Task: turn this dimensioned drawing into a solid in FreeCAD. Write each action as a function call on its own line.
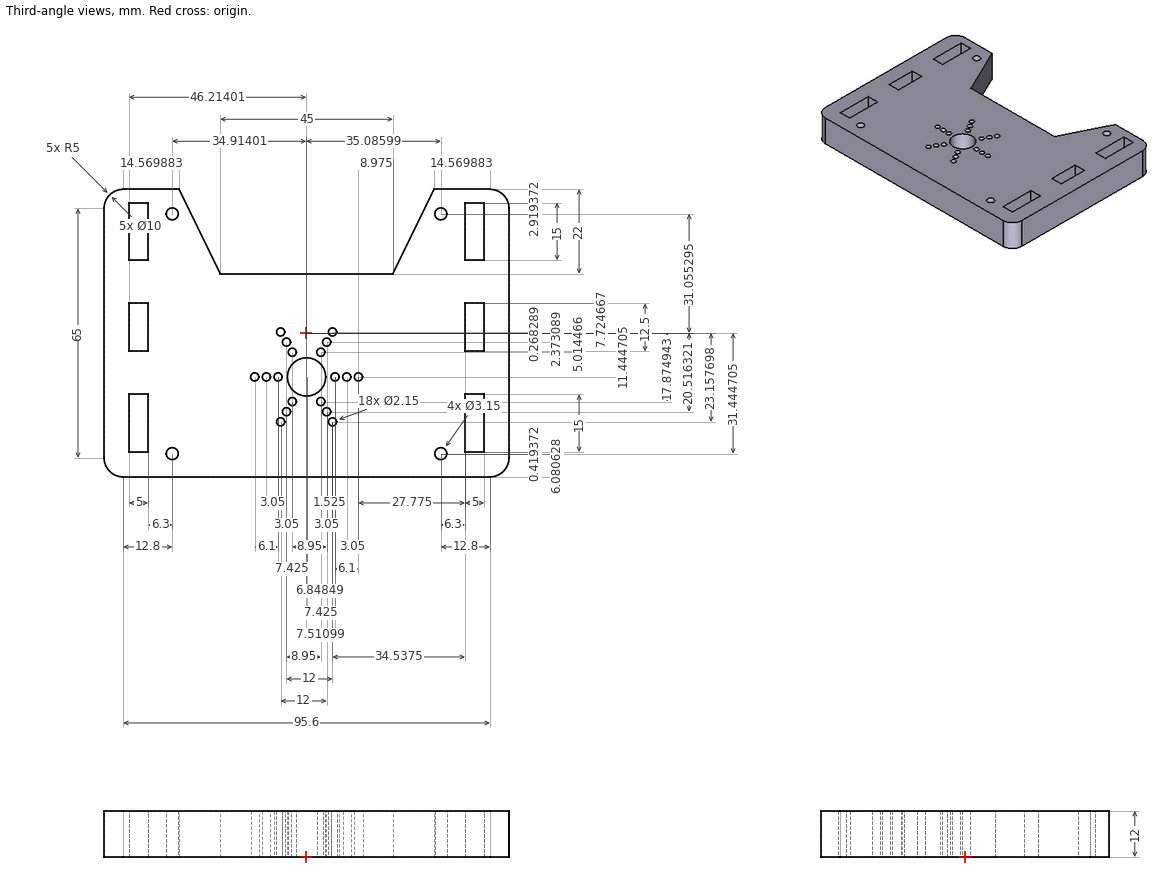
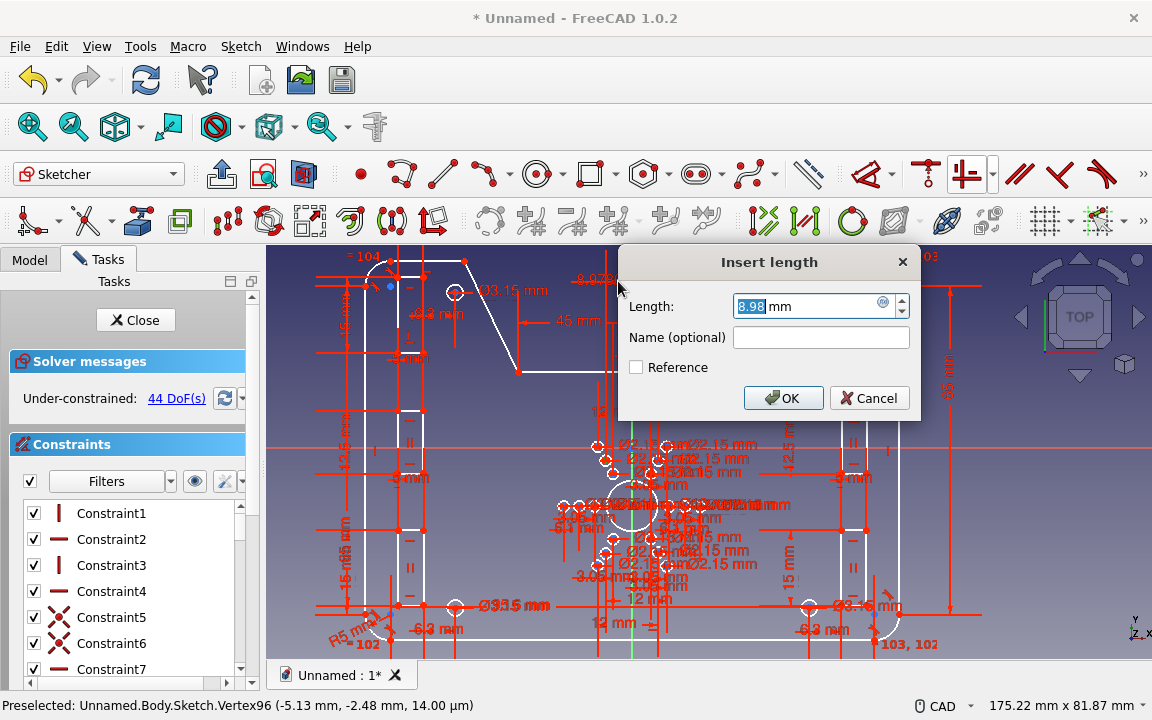
text(8.95)
key(Return)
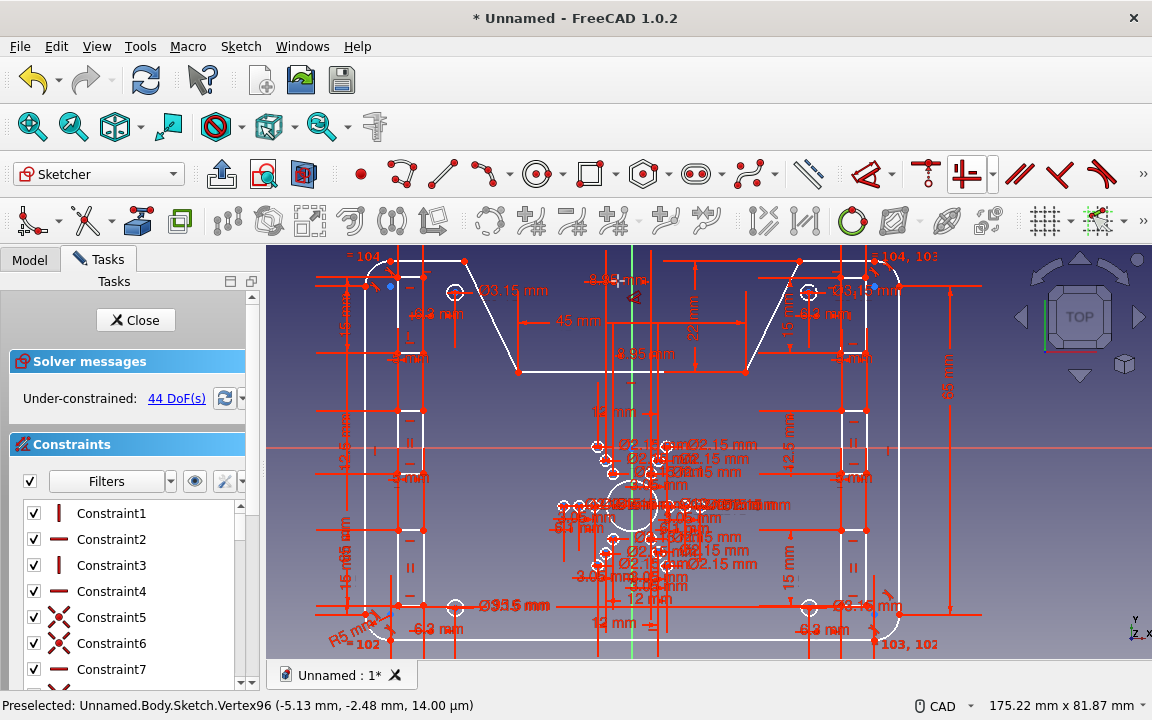
scroll(667, 566, up, 9)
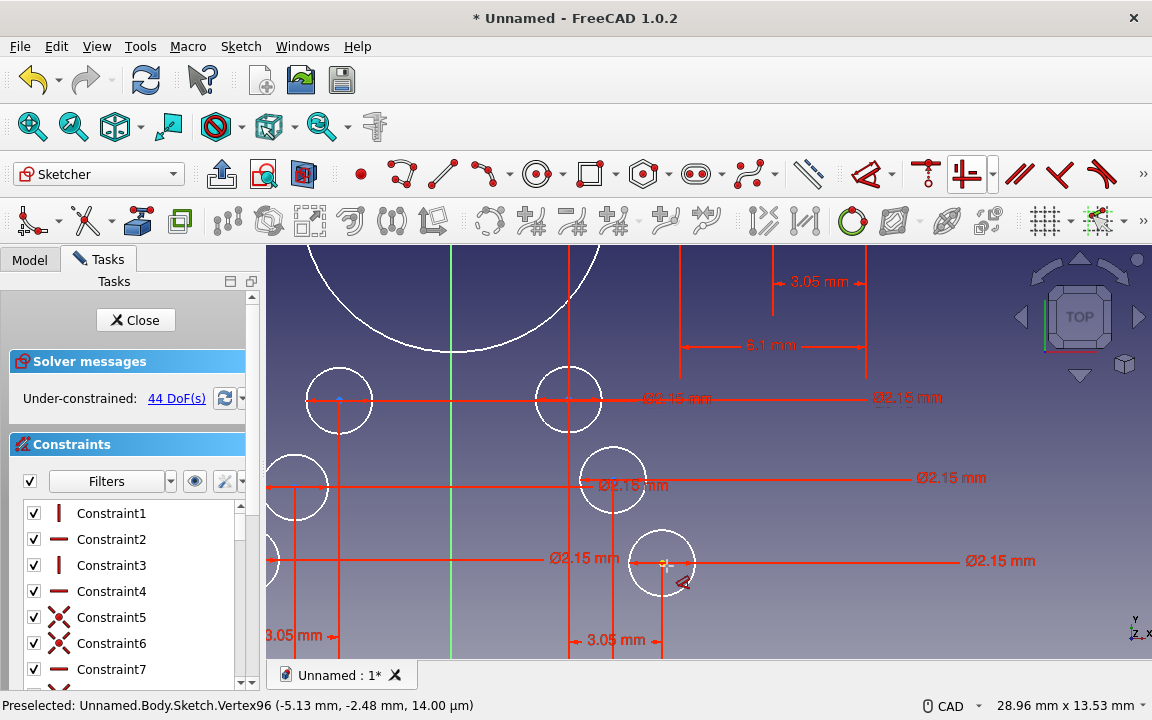
click(662, 563)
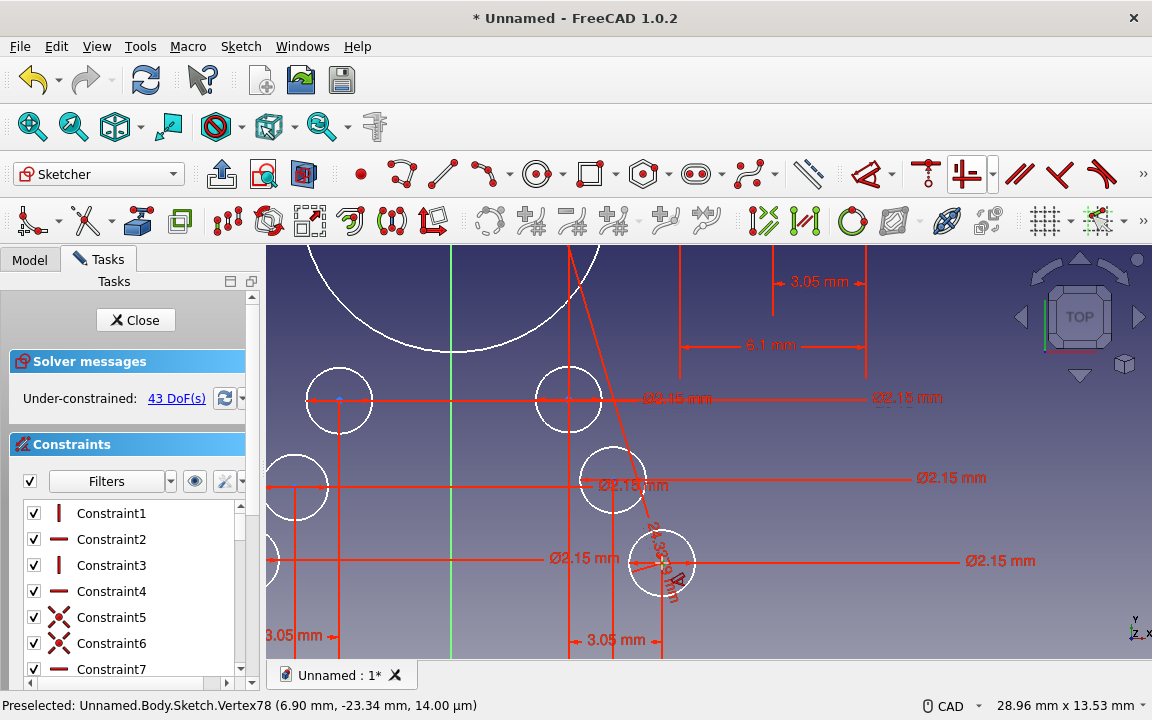
click(613, 480)
click(626, 597)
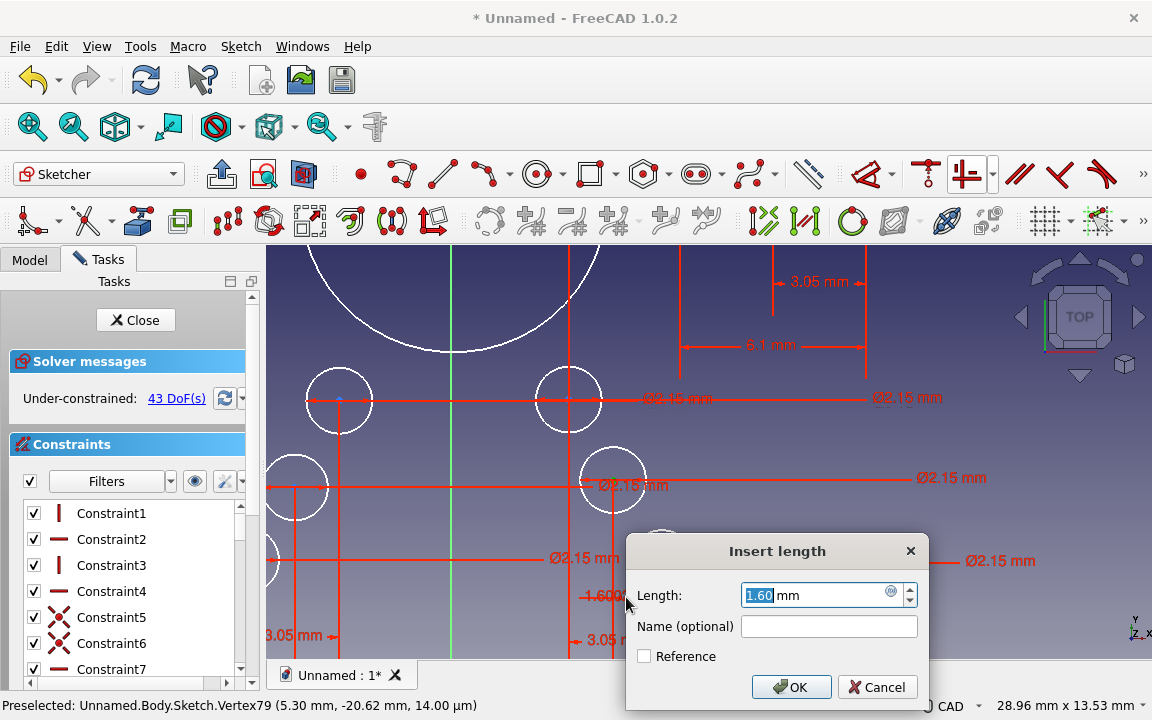
text(1.525)
key(Return)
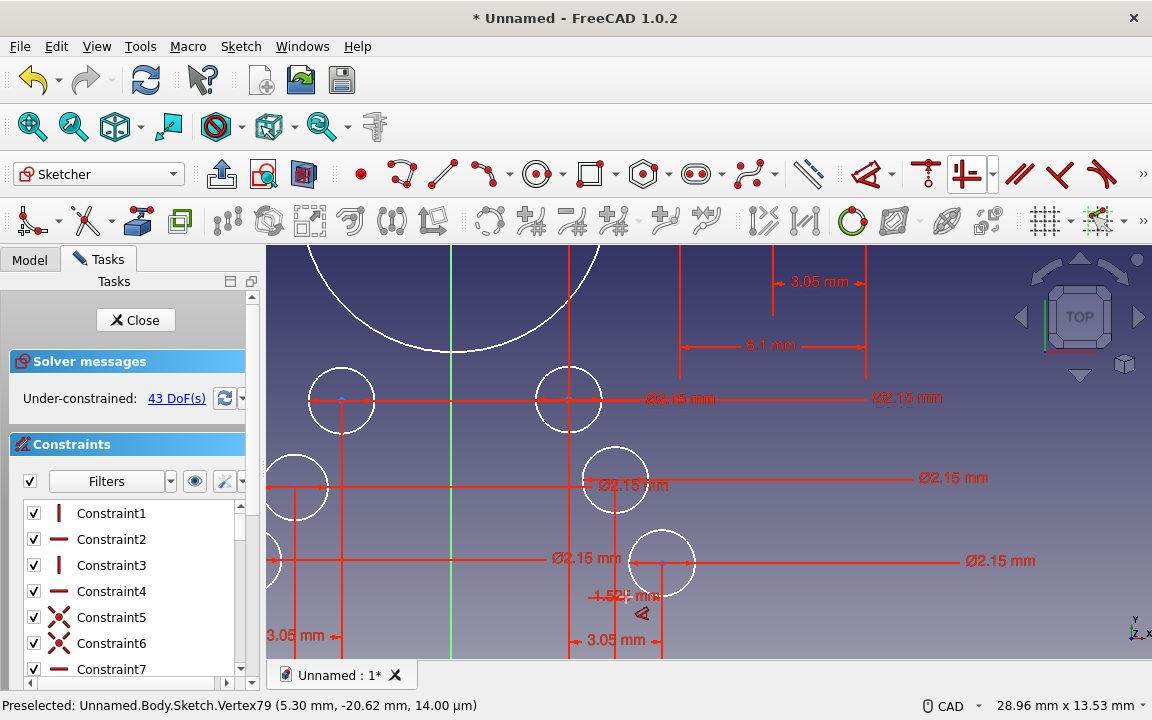
scroll(664, 527, down, 11)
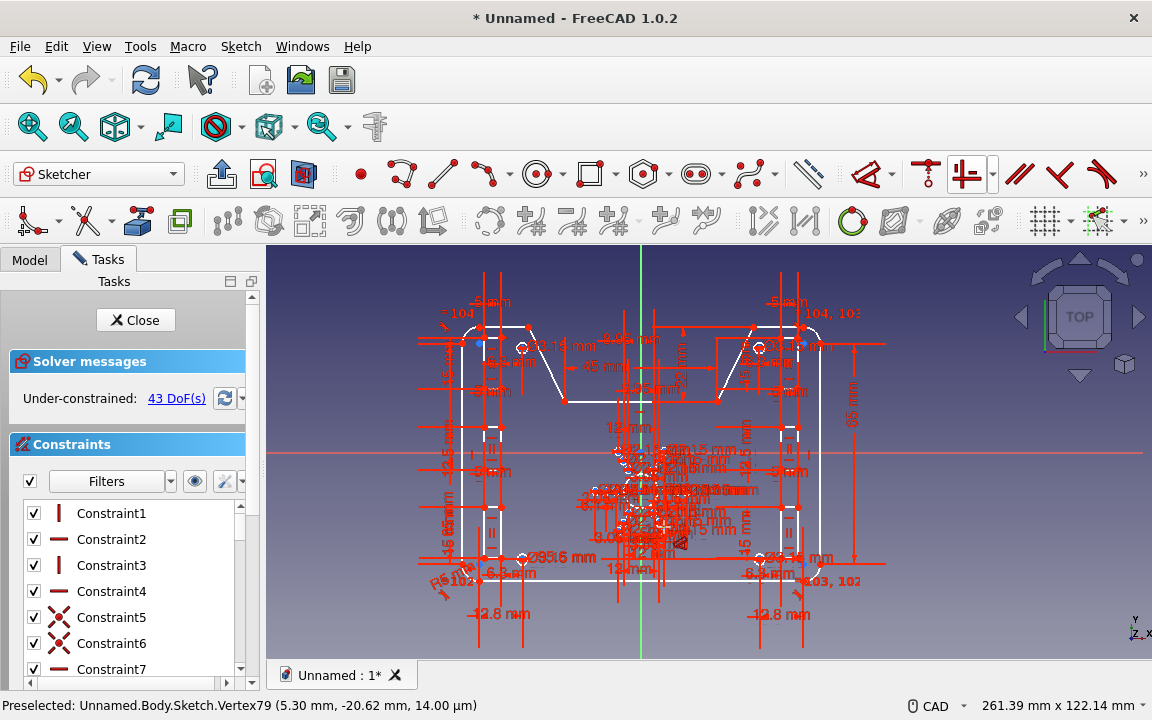
scroll(717, 402, up, 2)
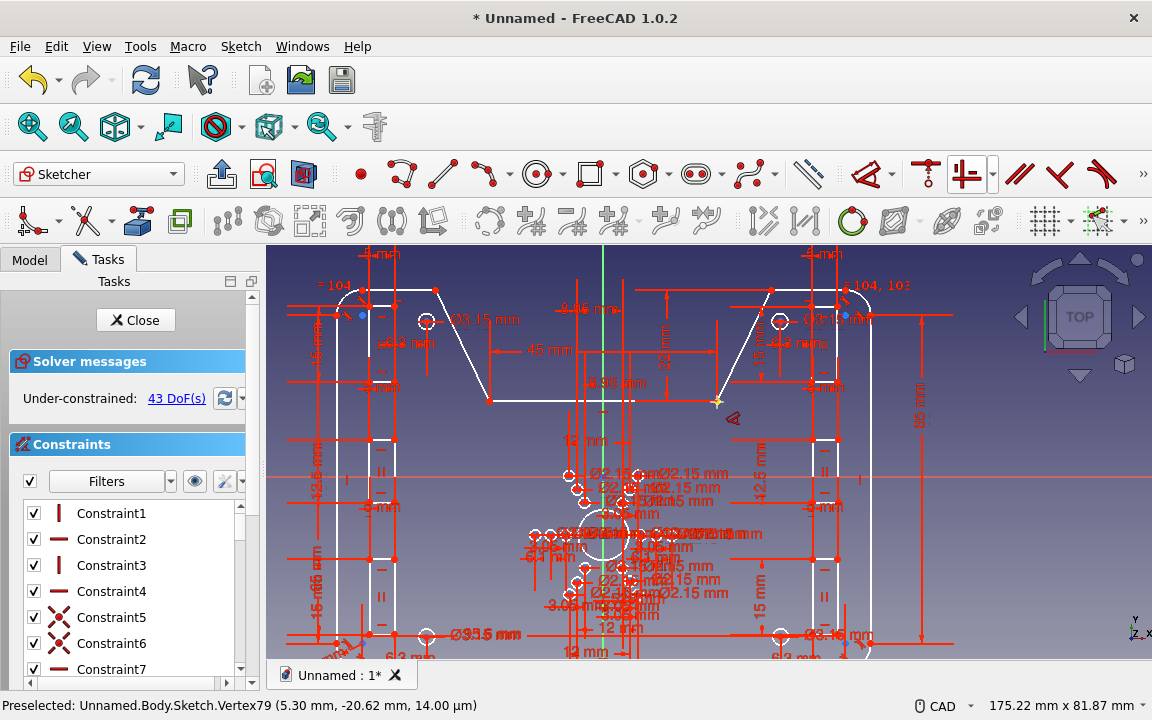
click(717, 401)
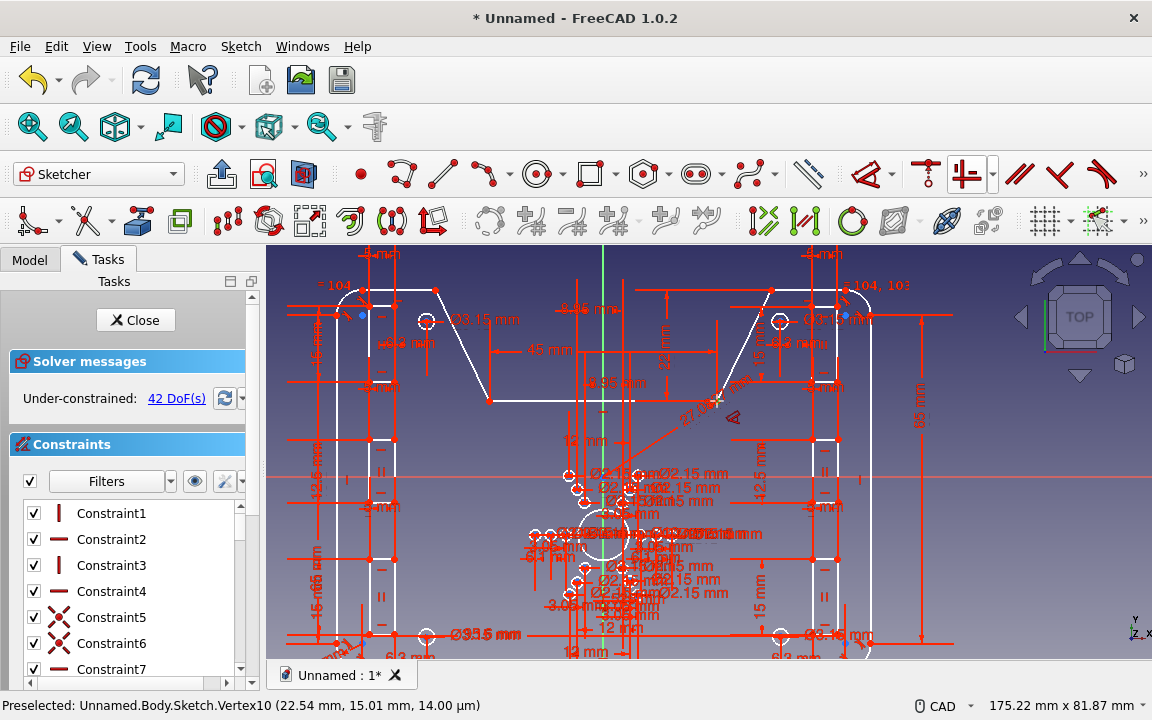
click(672, 536)
click(694, 367)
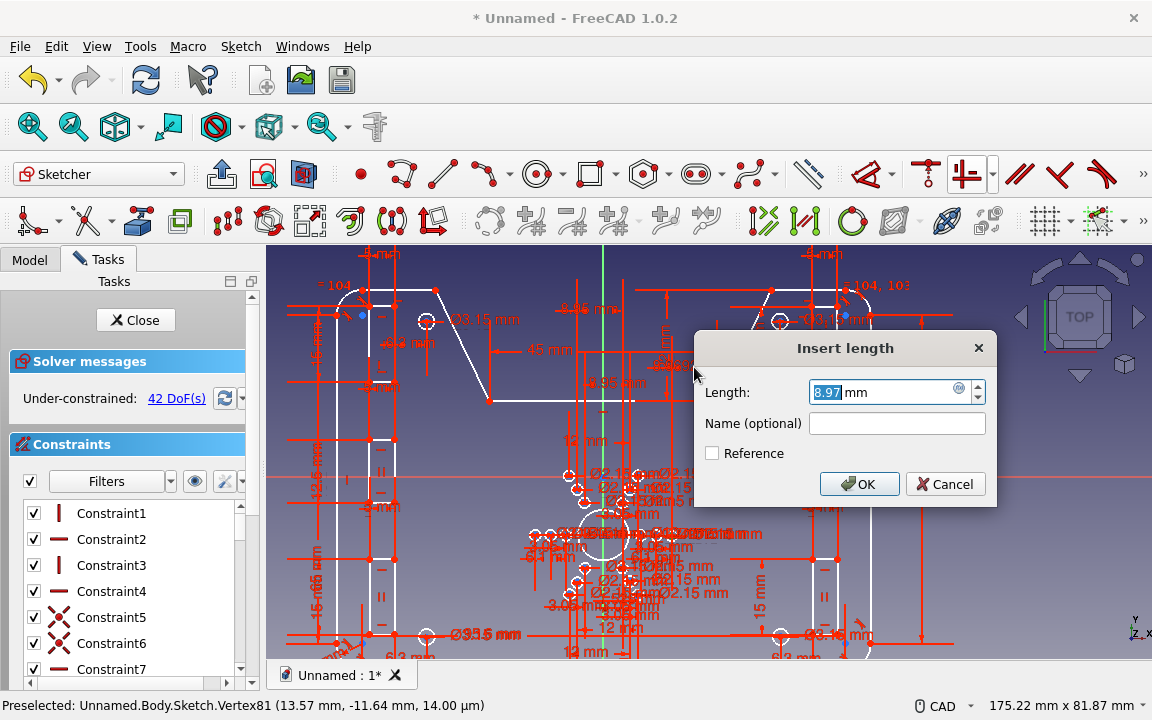
text(8.975)
key(Return)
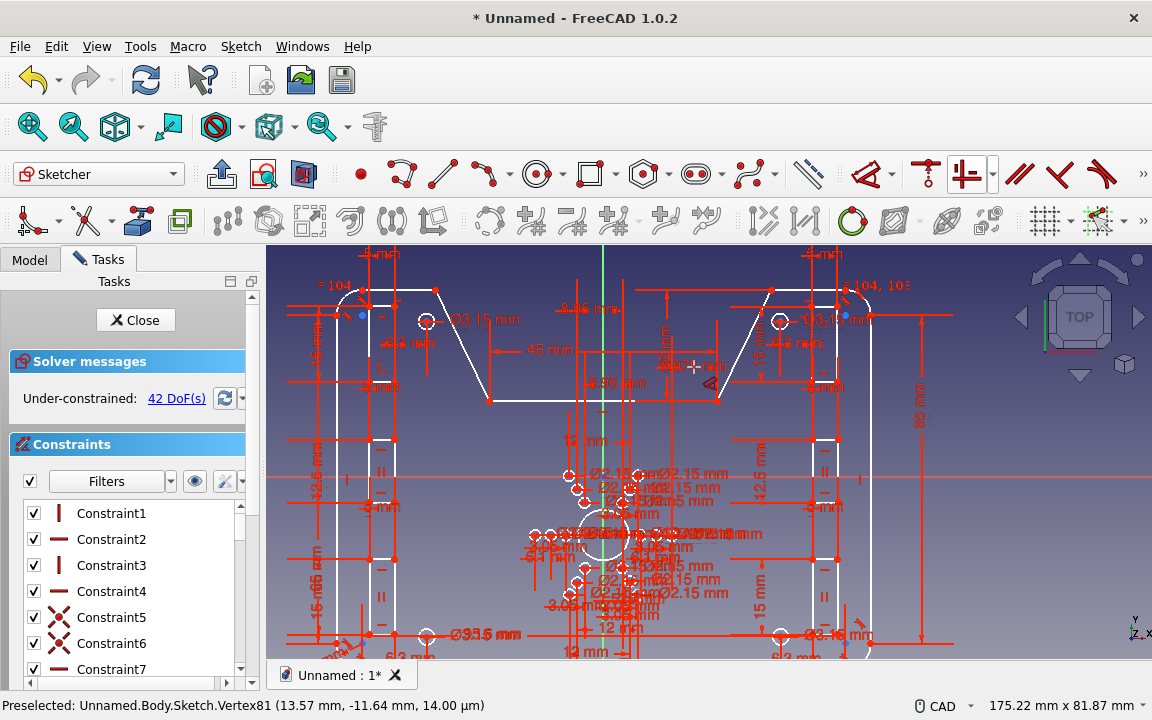
scroll(638, 476, up, 9)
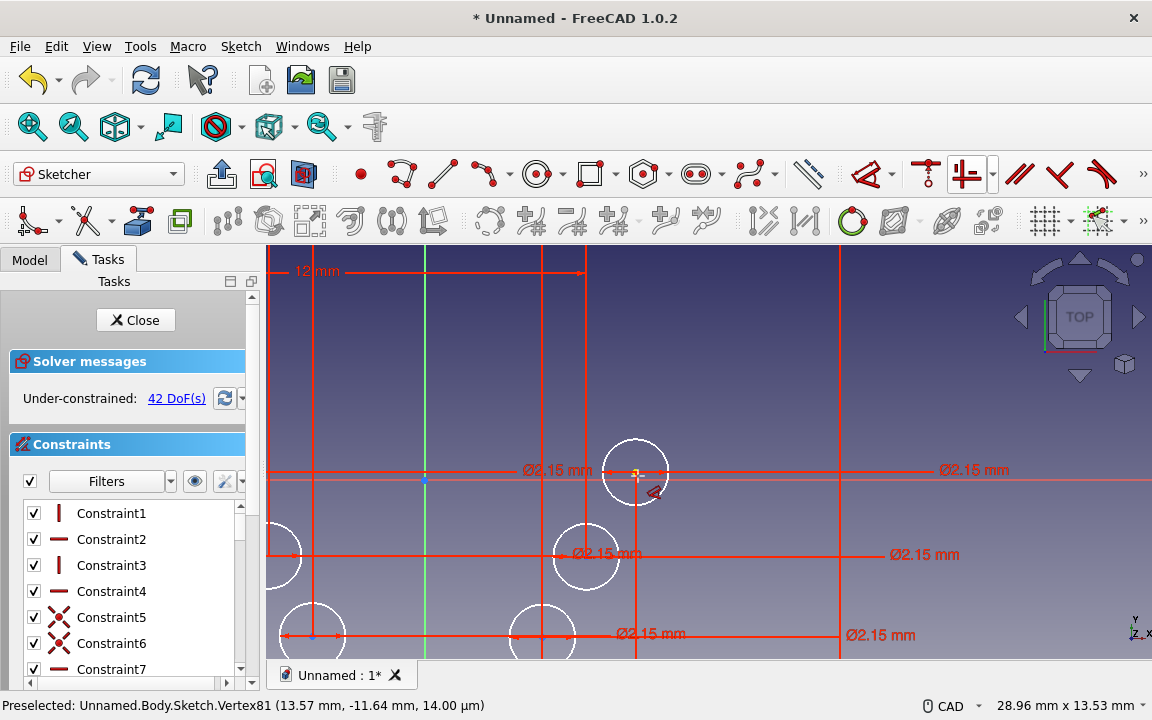
click(636, 472)